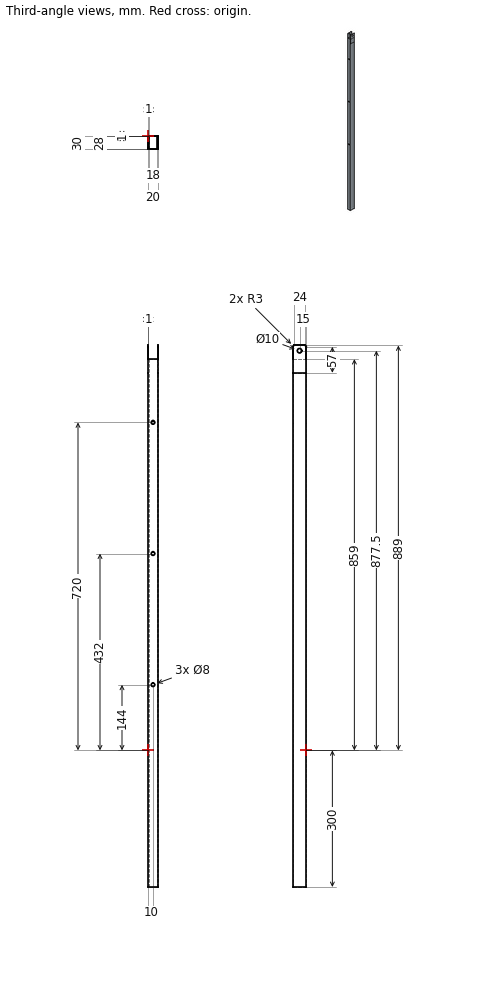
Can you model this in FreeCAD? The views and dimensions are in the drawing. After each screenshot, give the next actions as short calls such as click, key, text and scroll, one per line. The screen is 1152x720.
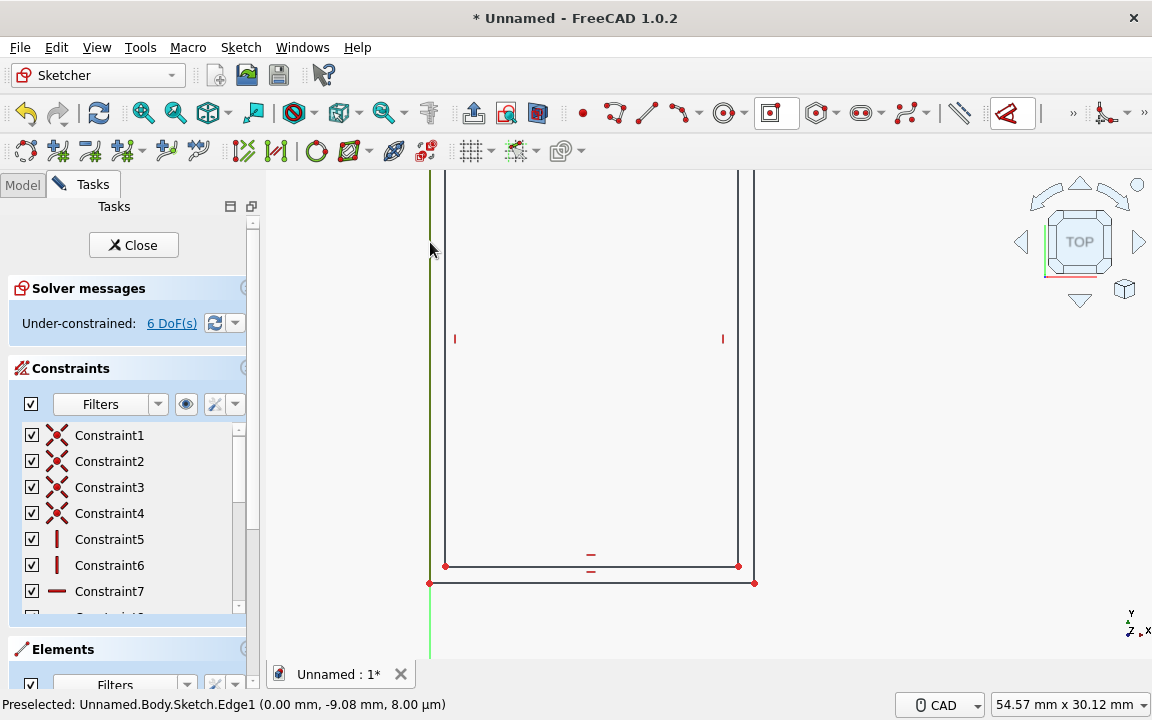
key(i)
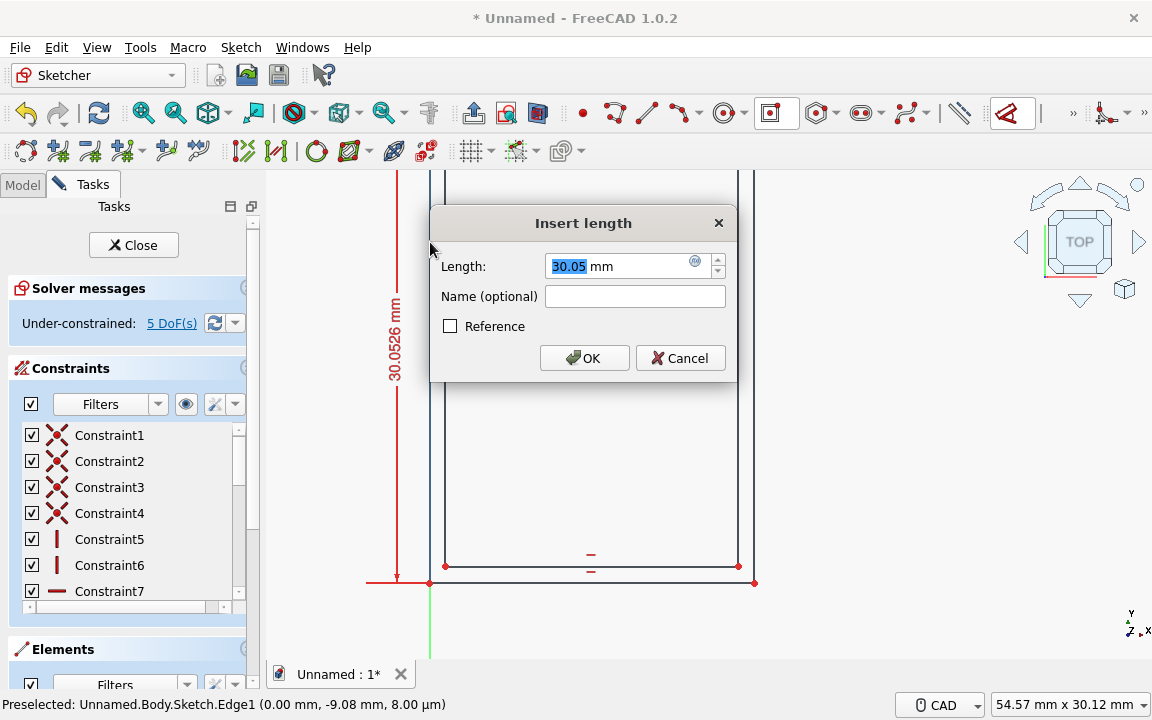
text(30)
key(Return)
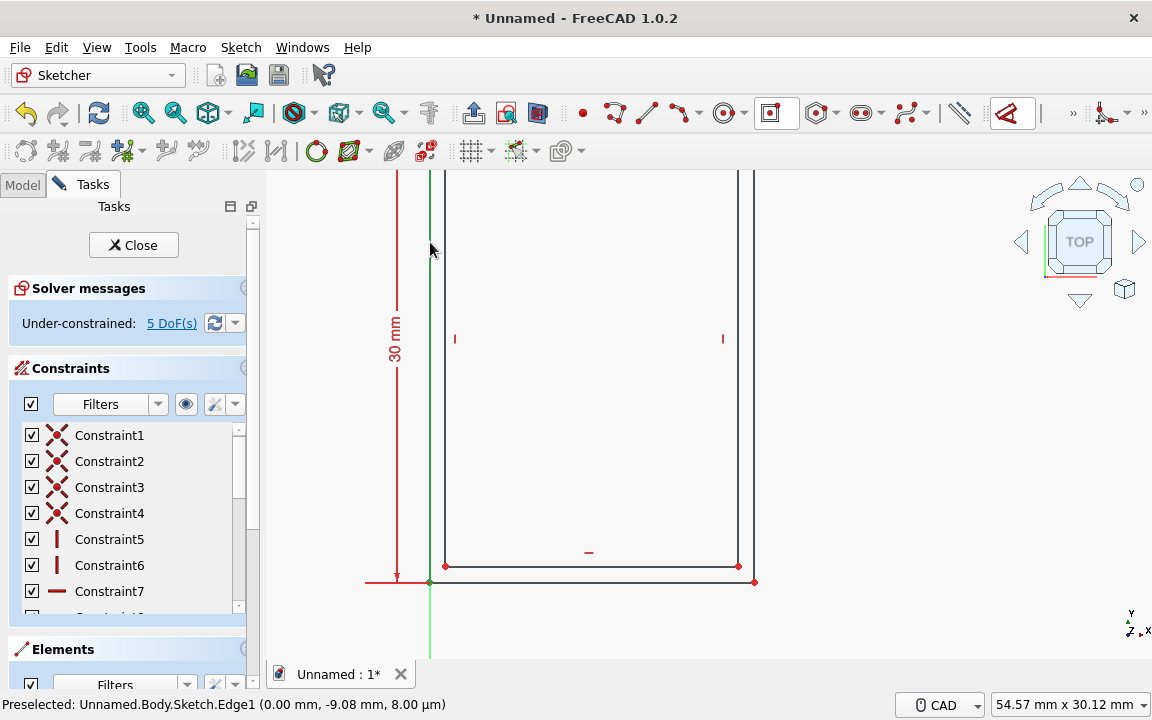
click(527, 583)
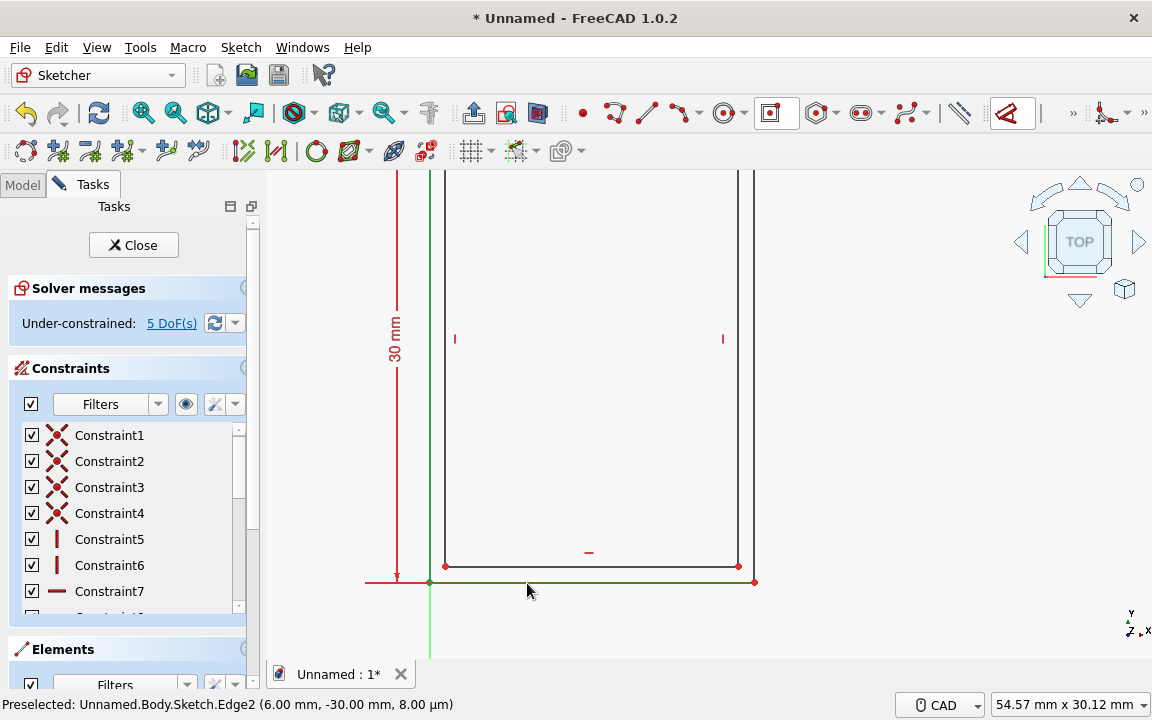
click(1030, 114)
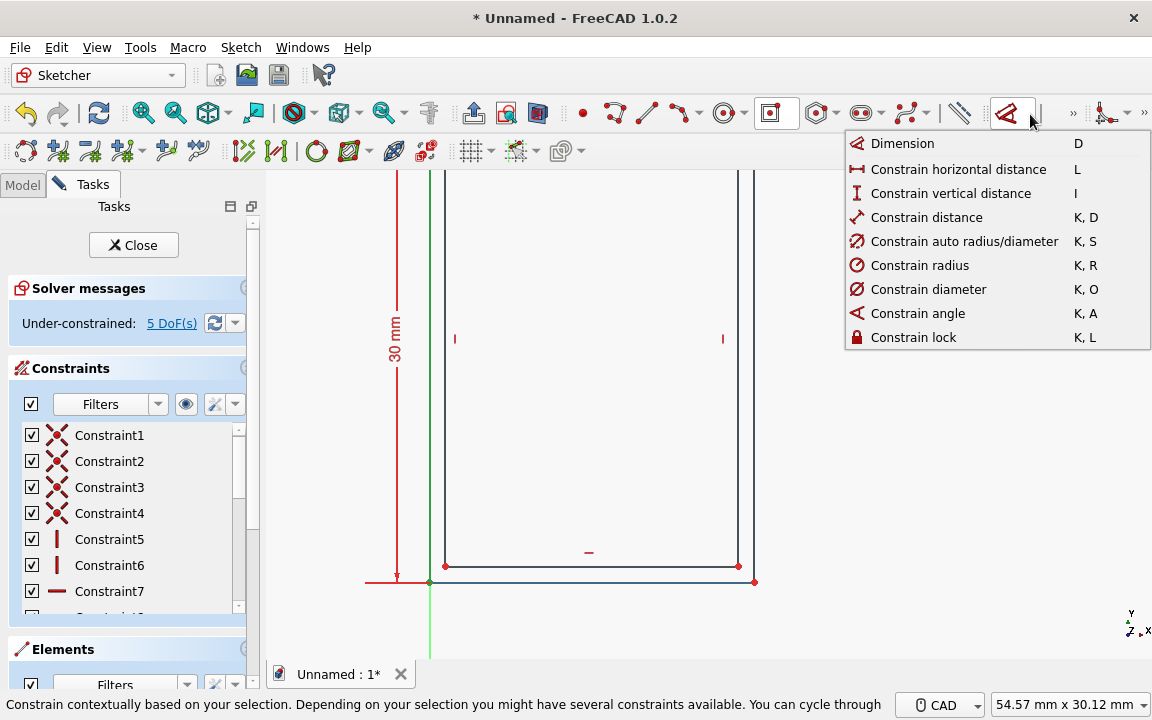
click(998, 169)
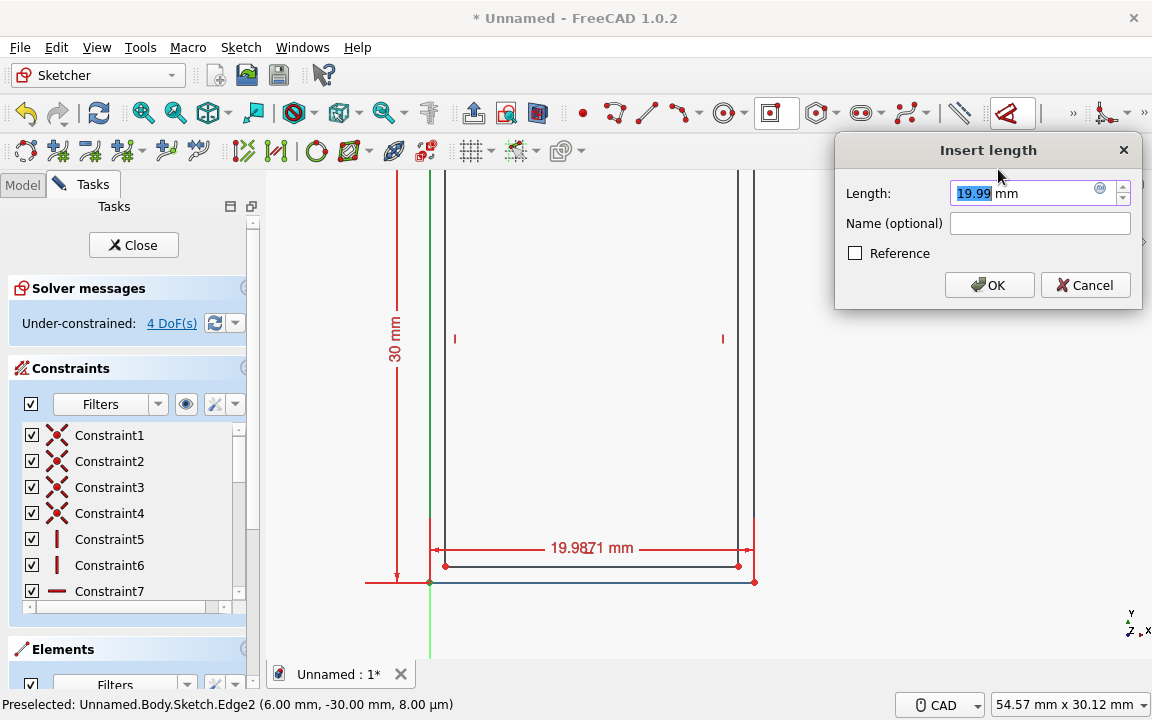
text(20)
key(Return)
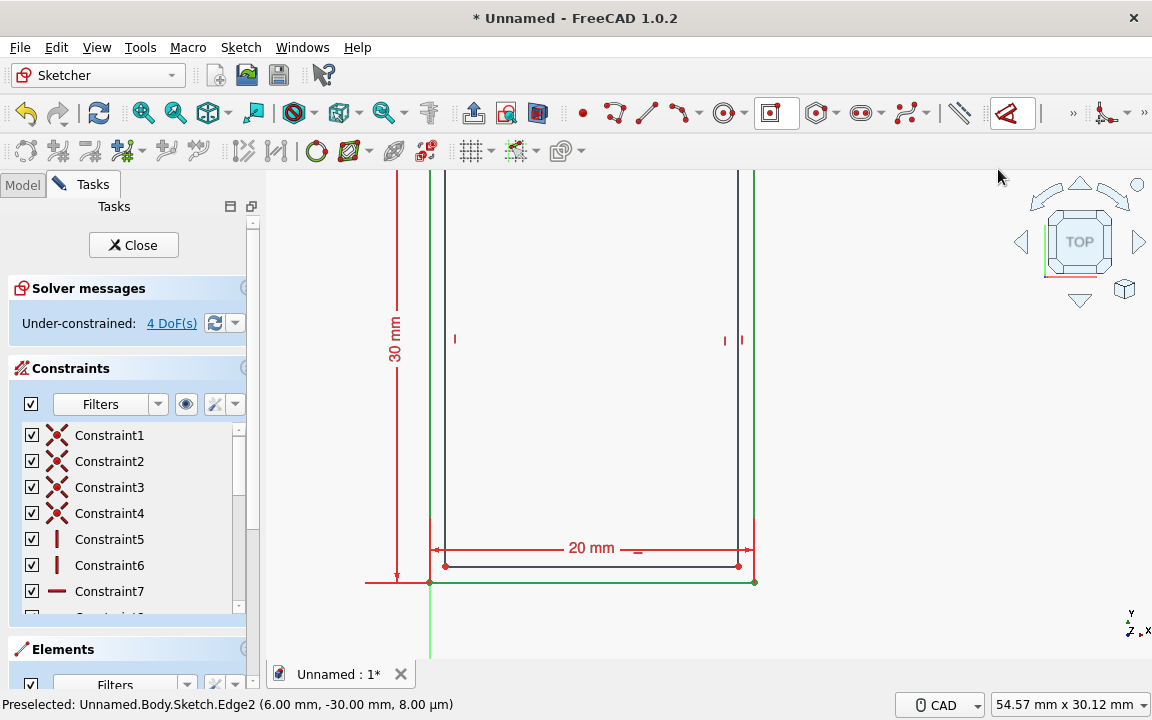
click(445, 249)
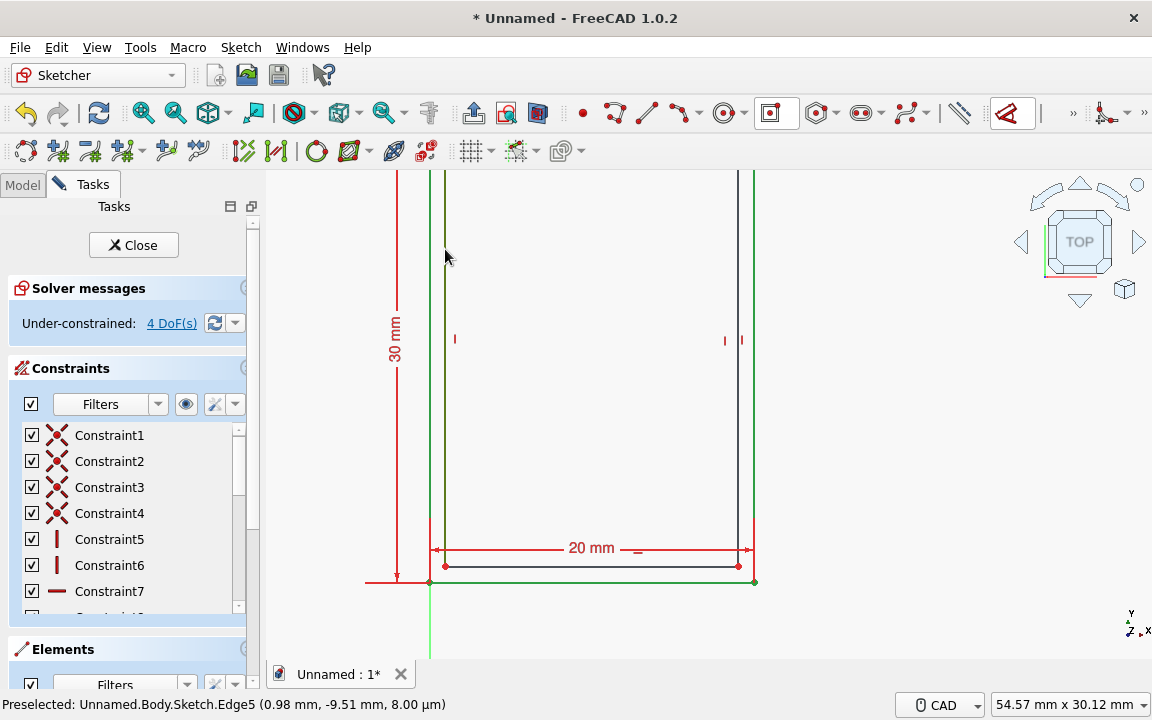
key(i)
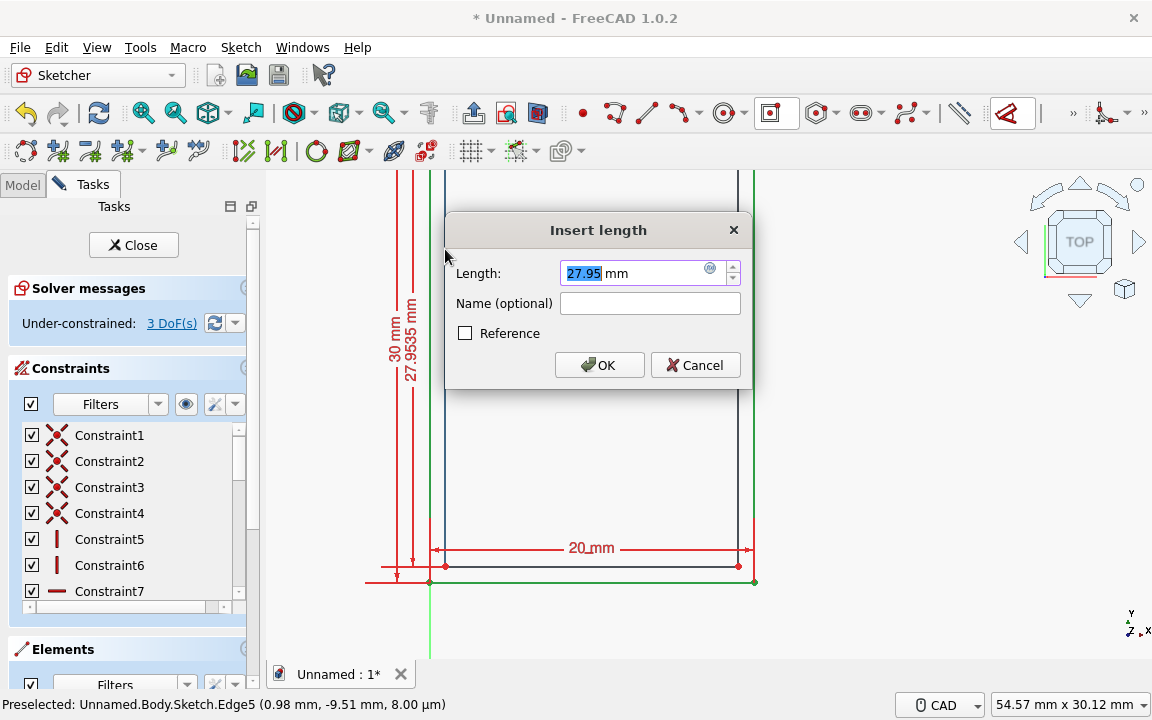
text(28)
key(Return)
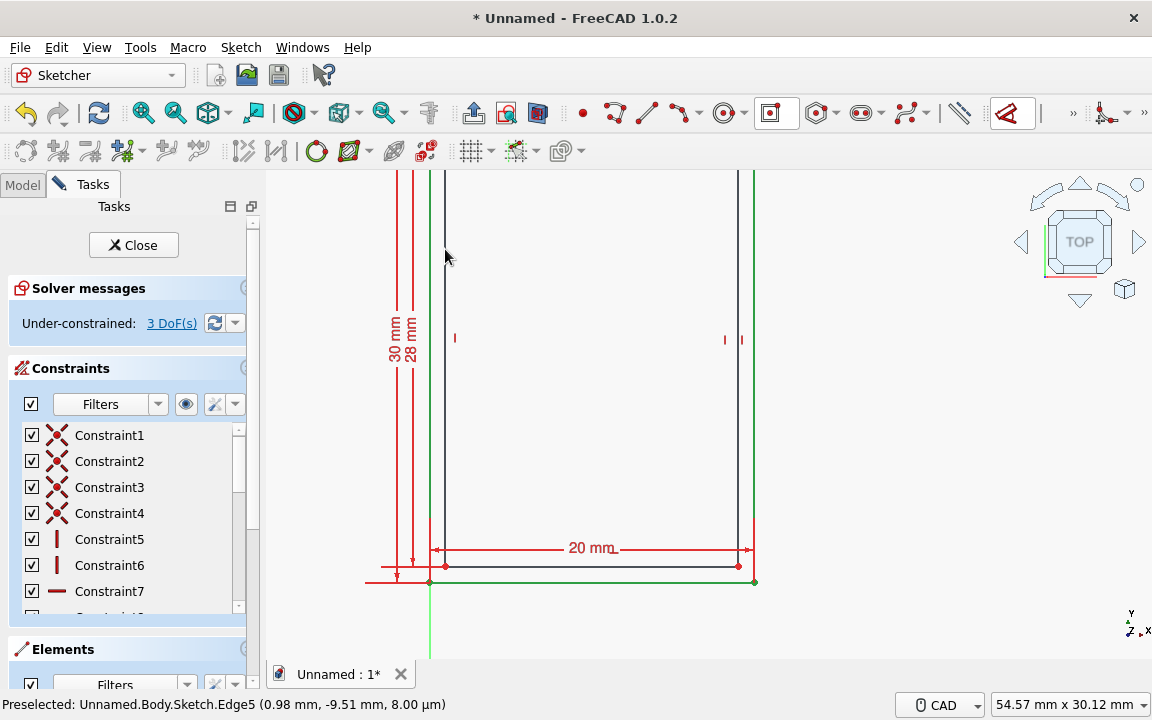
click(533, 567)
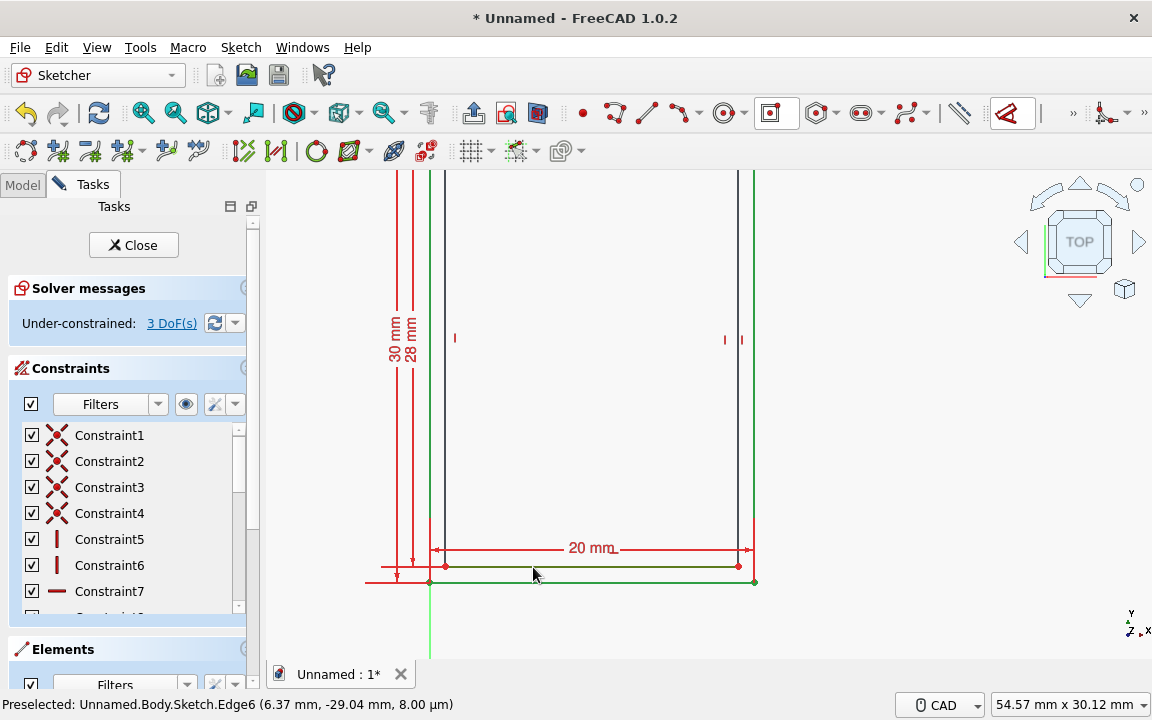
key(l)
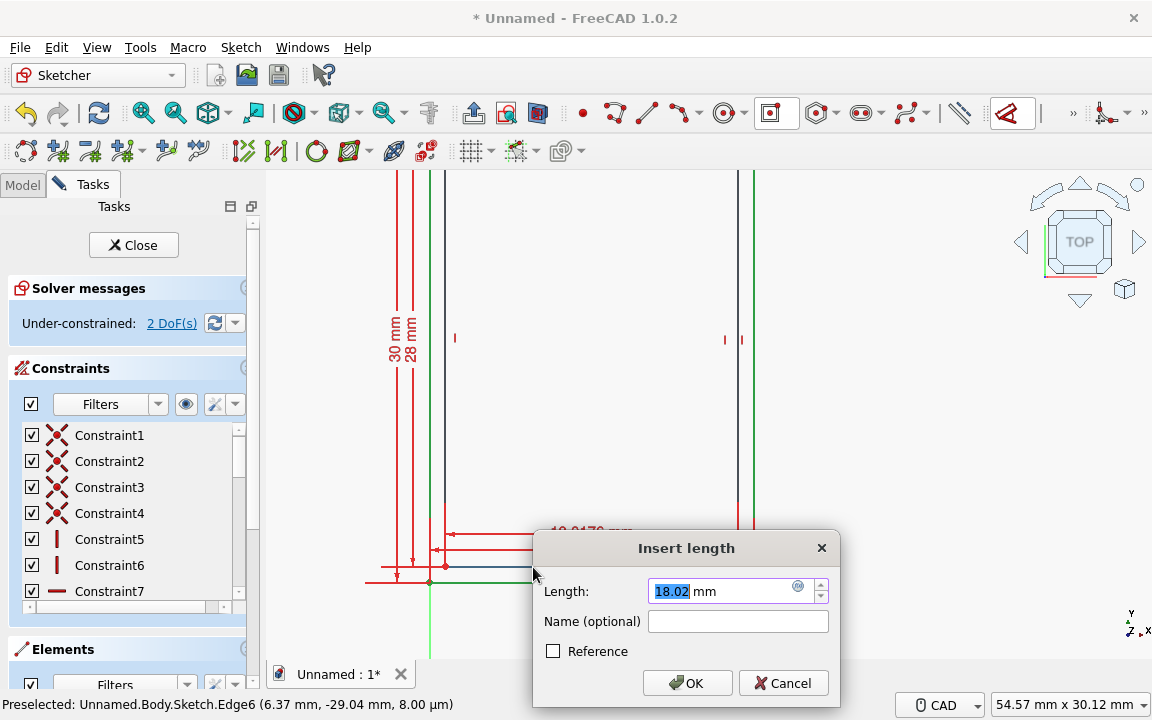
text(18)
key(Return)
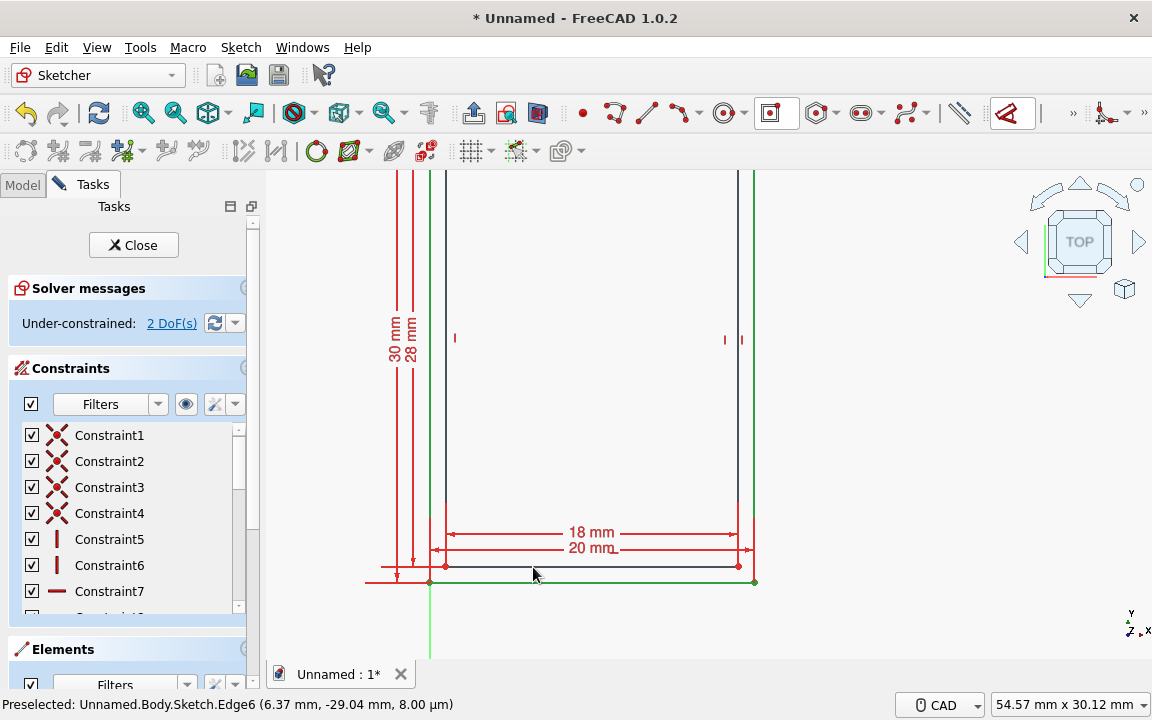
scroll(739, 568, down, 2)